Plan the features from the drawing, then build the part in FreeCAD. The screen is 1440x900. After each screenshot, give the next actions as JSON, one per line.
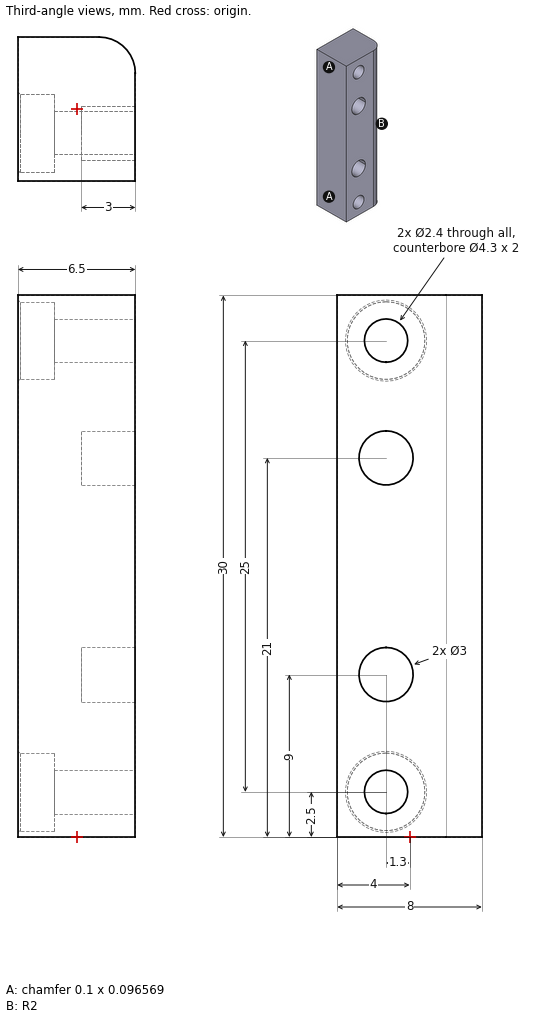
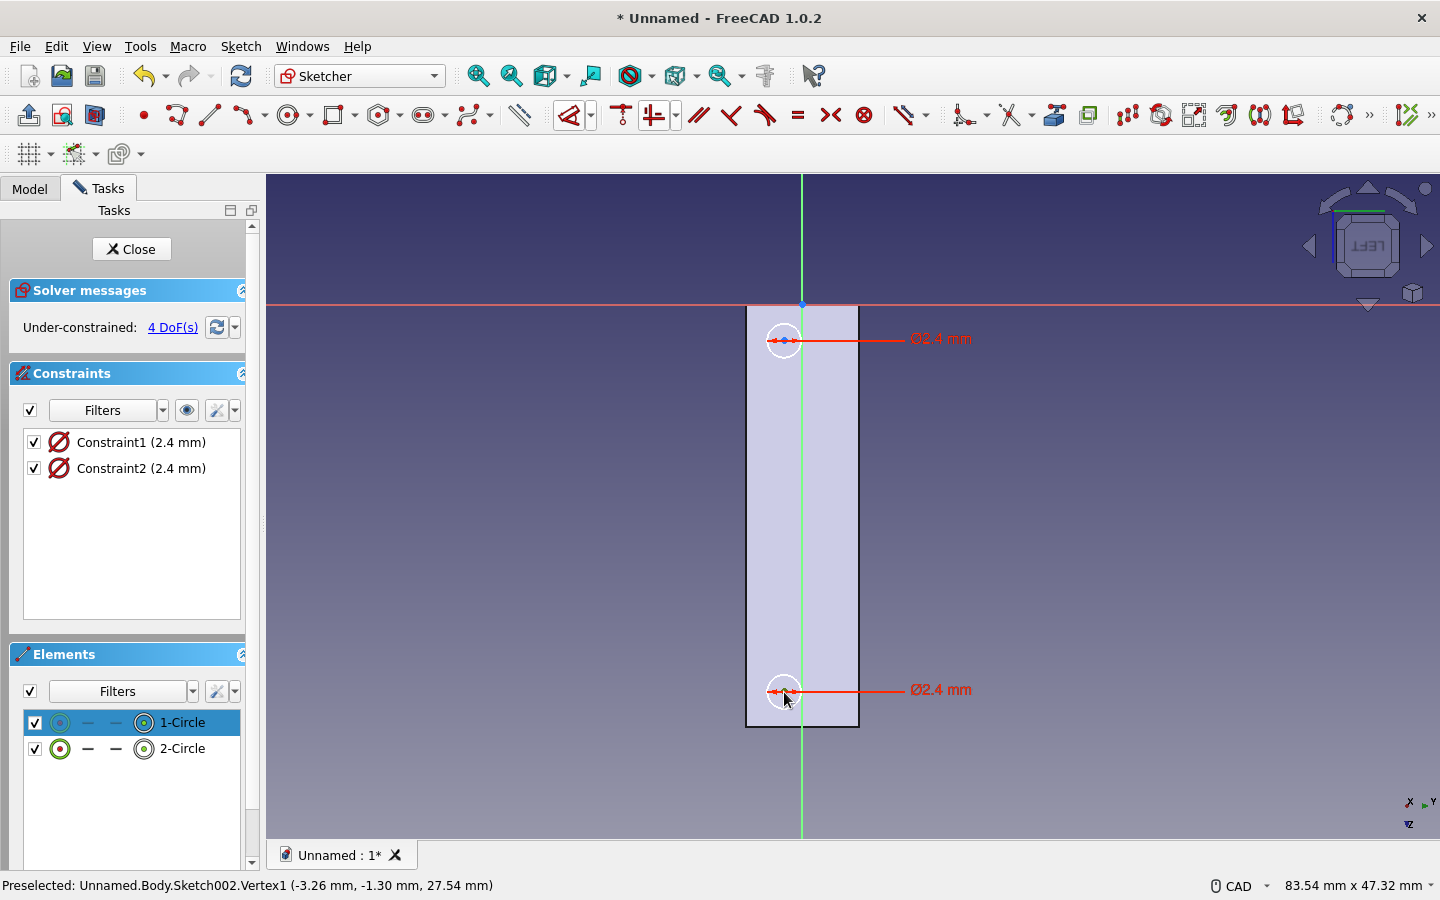
{"action": "left_click", "coordinate": [784, 341]}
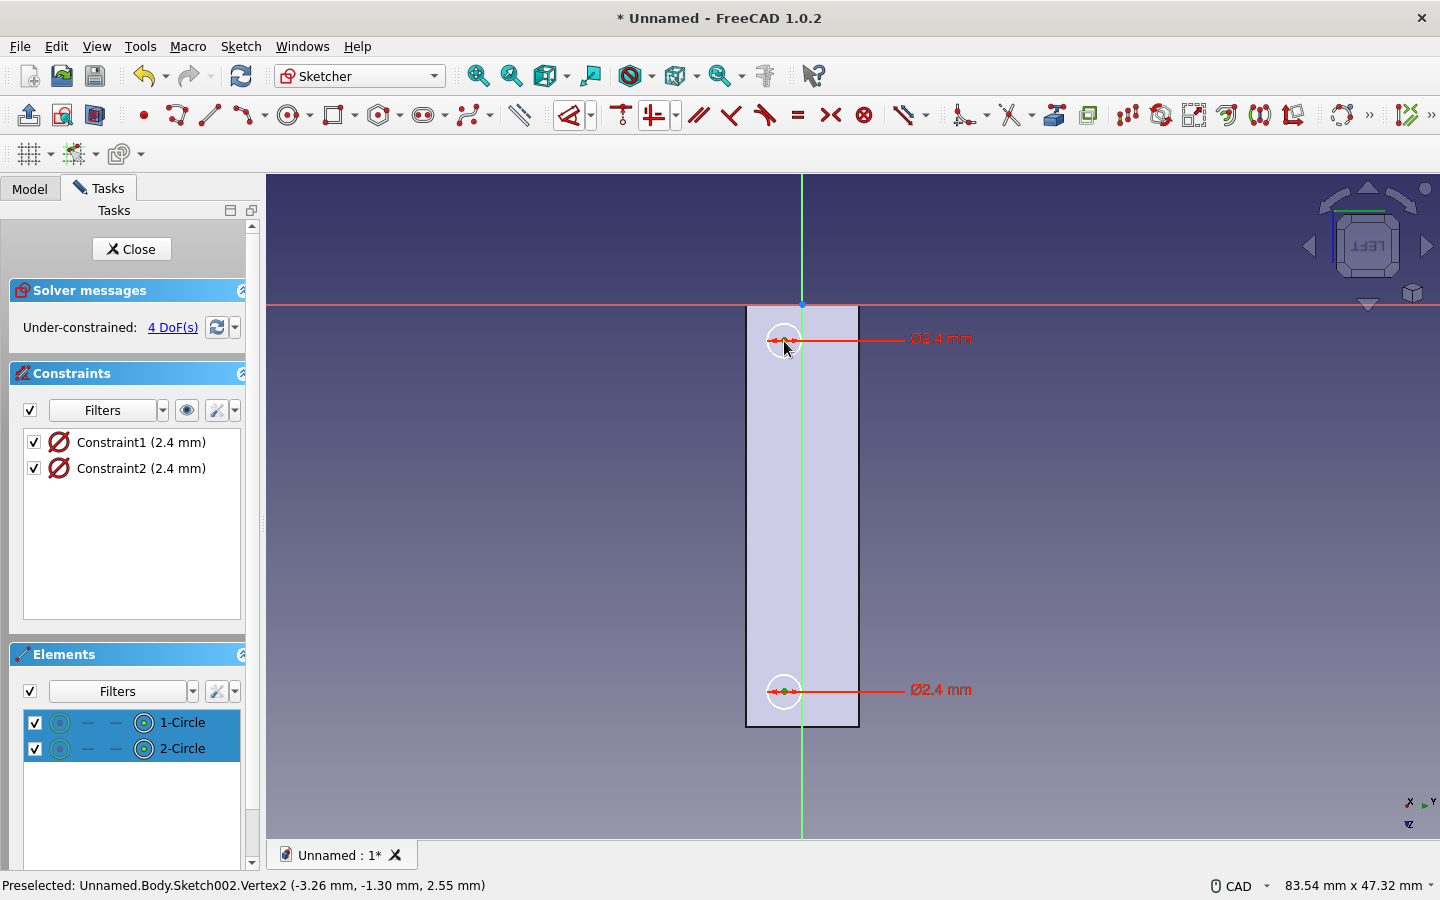
{"action": "key", "text": "v"}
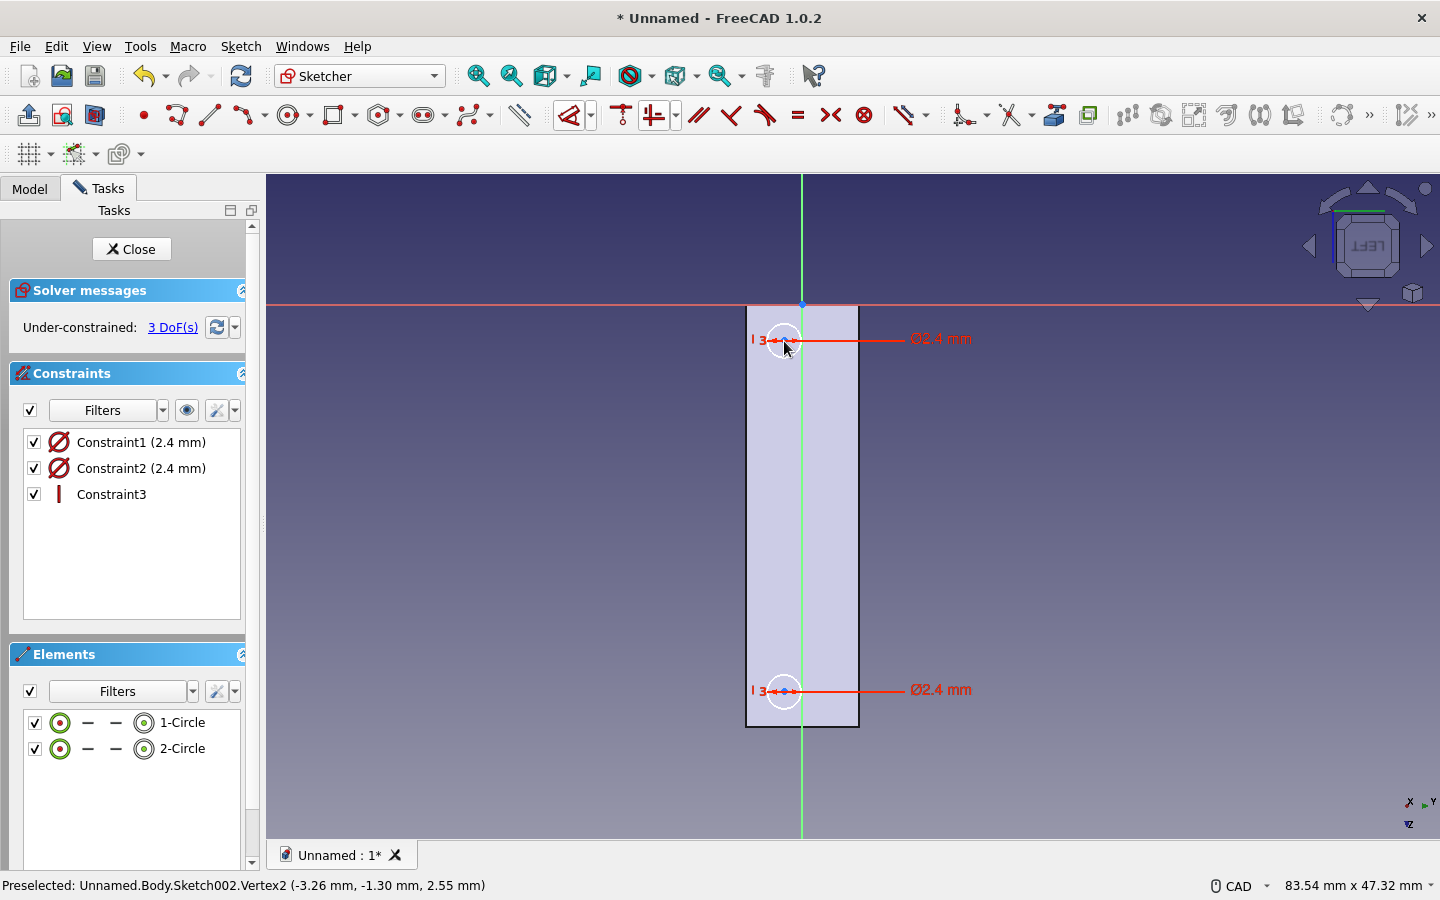
{"action": "scroll", "coordinate": [784, 692], "scroll_direction": "up", "scroll_amount": 4}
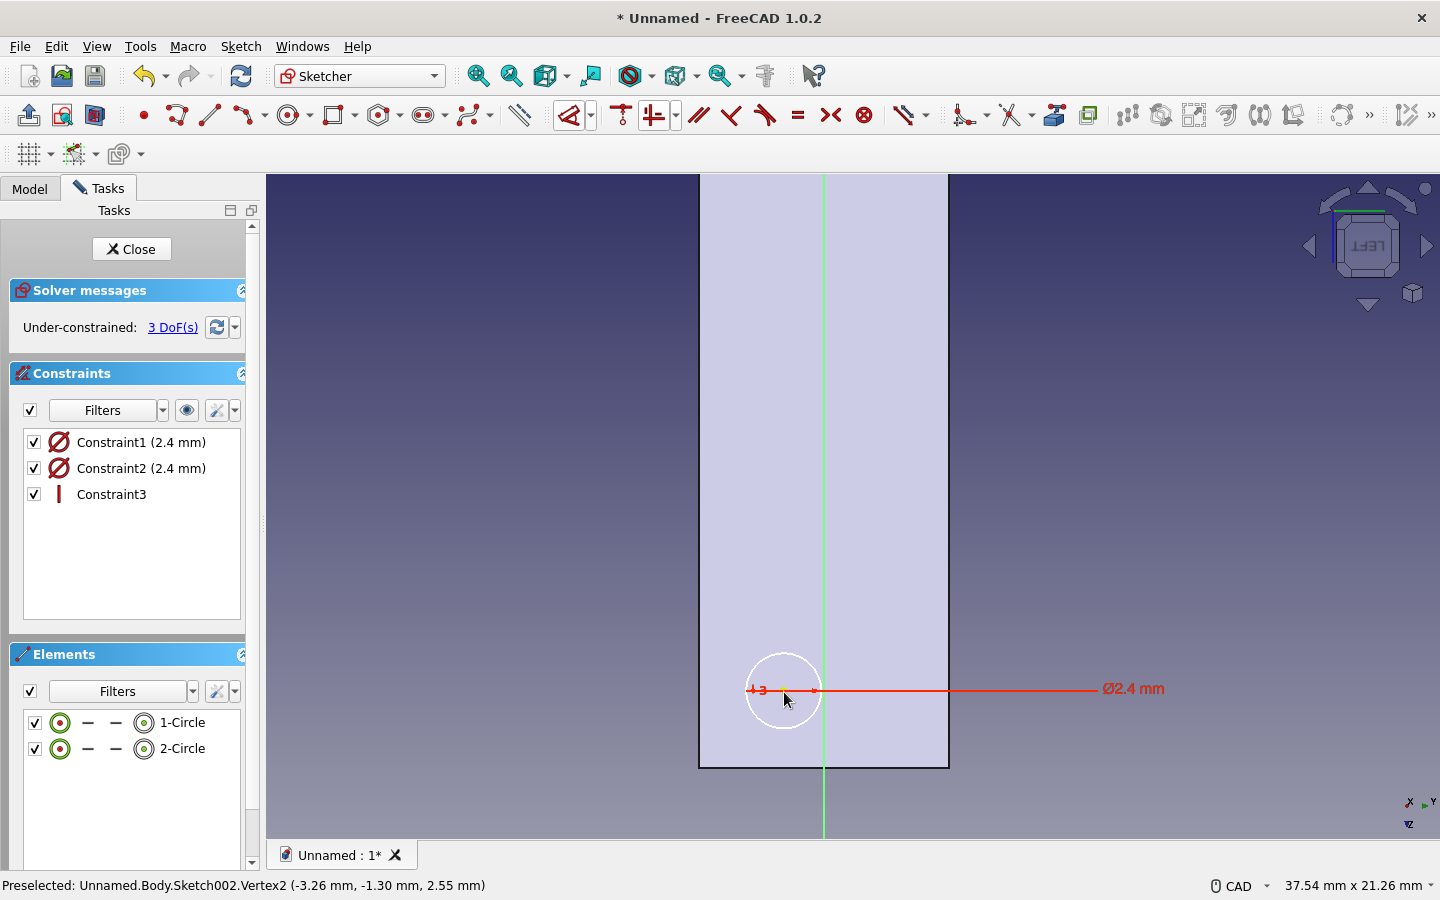
{"action": "left_click", "coordinate": [784, 691]}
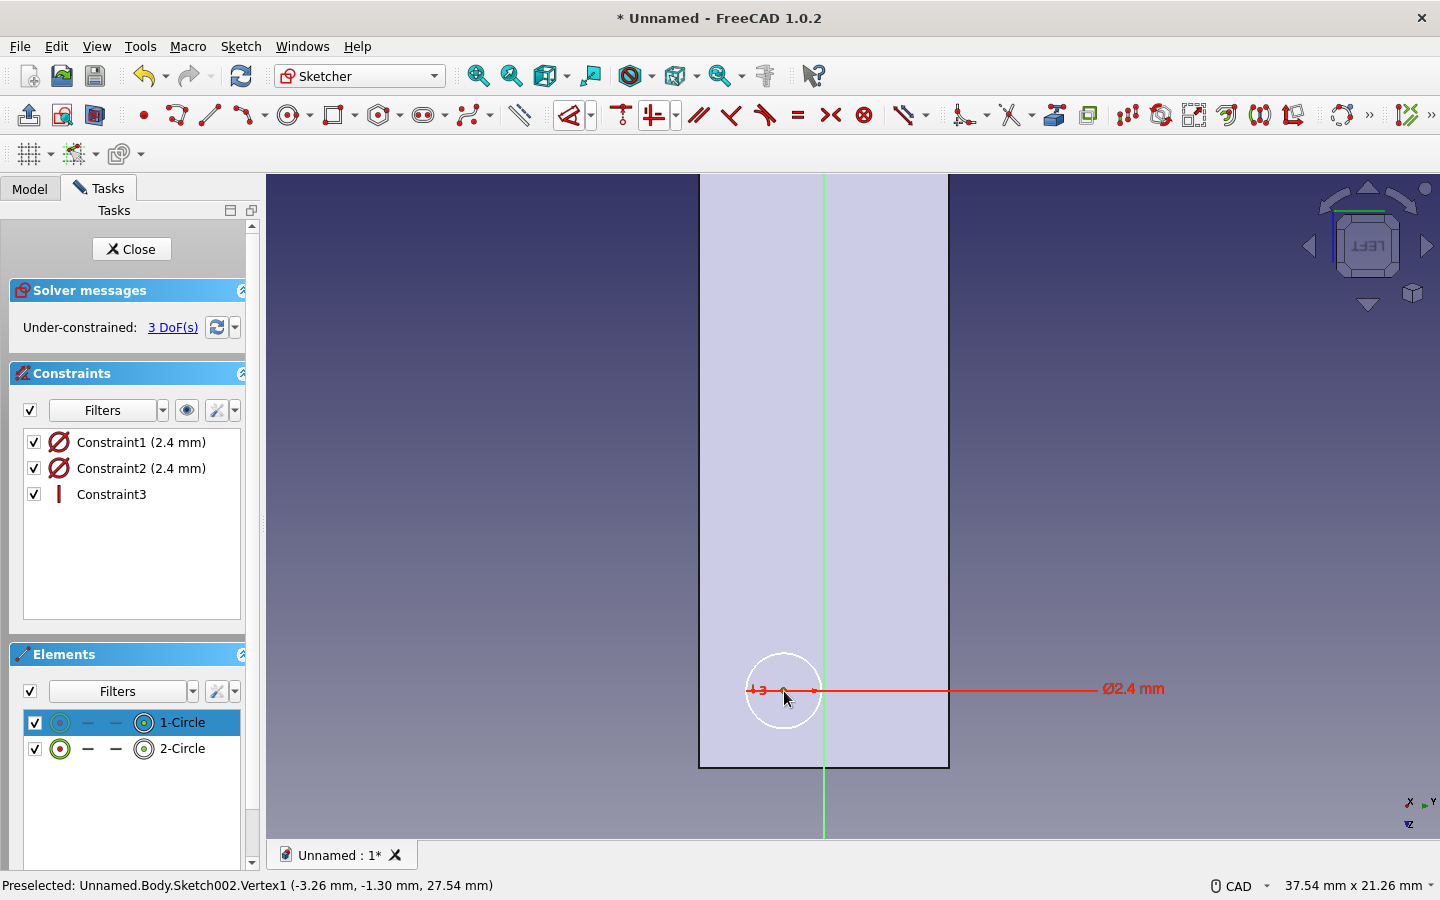
{"action": "left_click", "coordinate": [590, 116]}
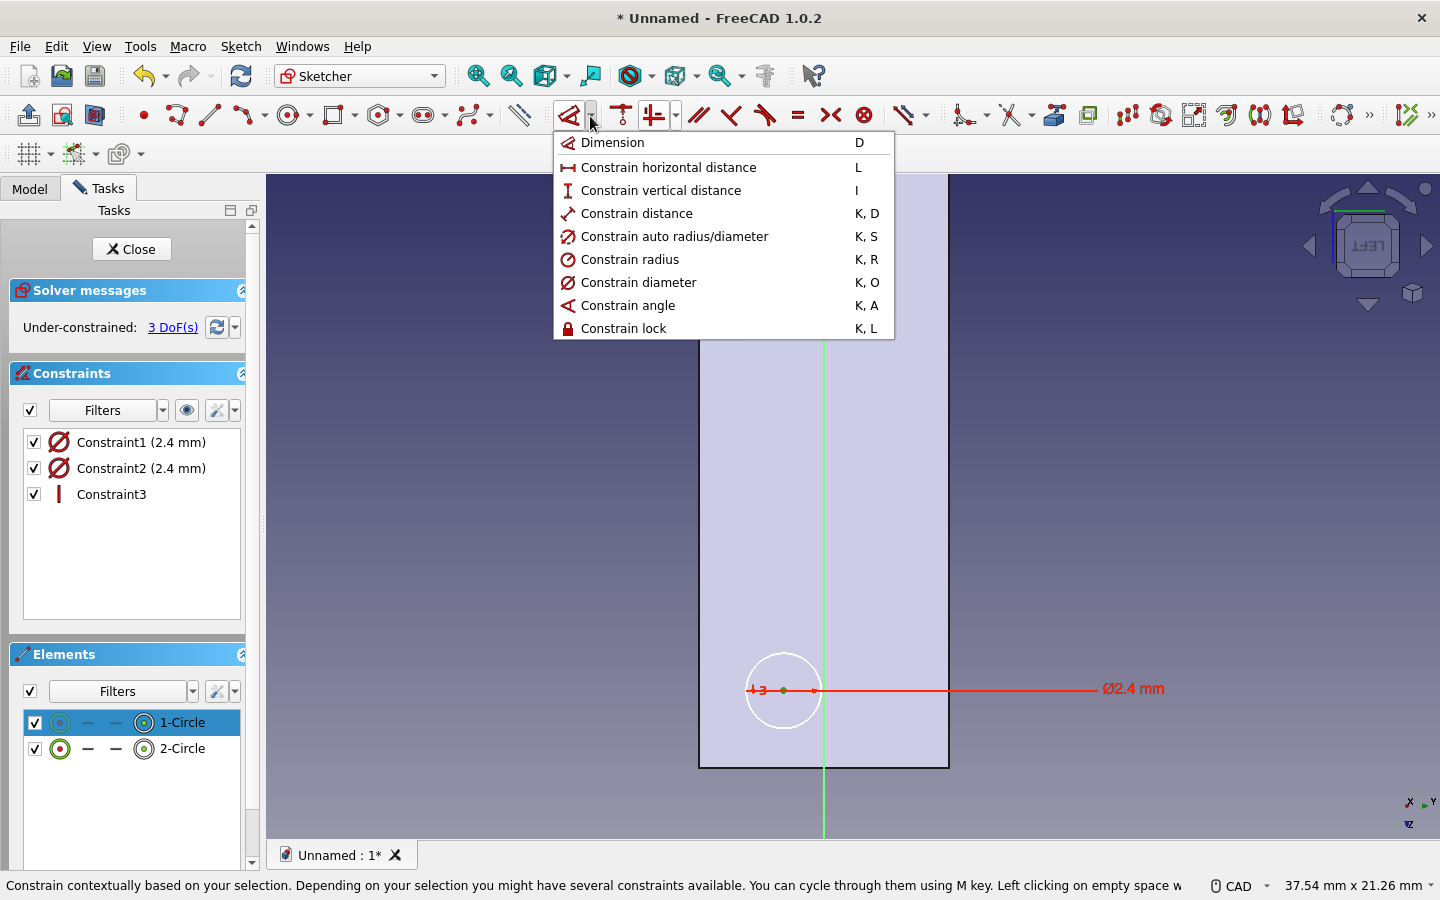
{"action": "left_click", "coordinate": [724, 168]}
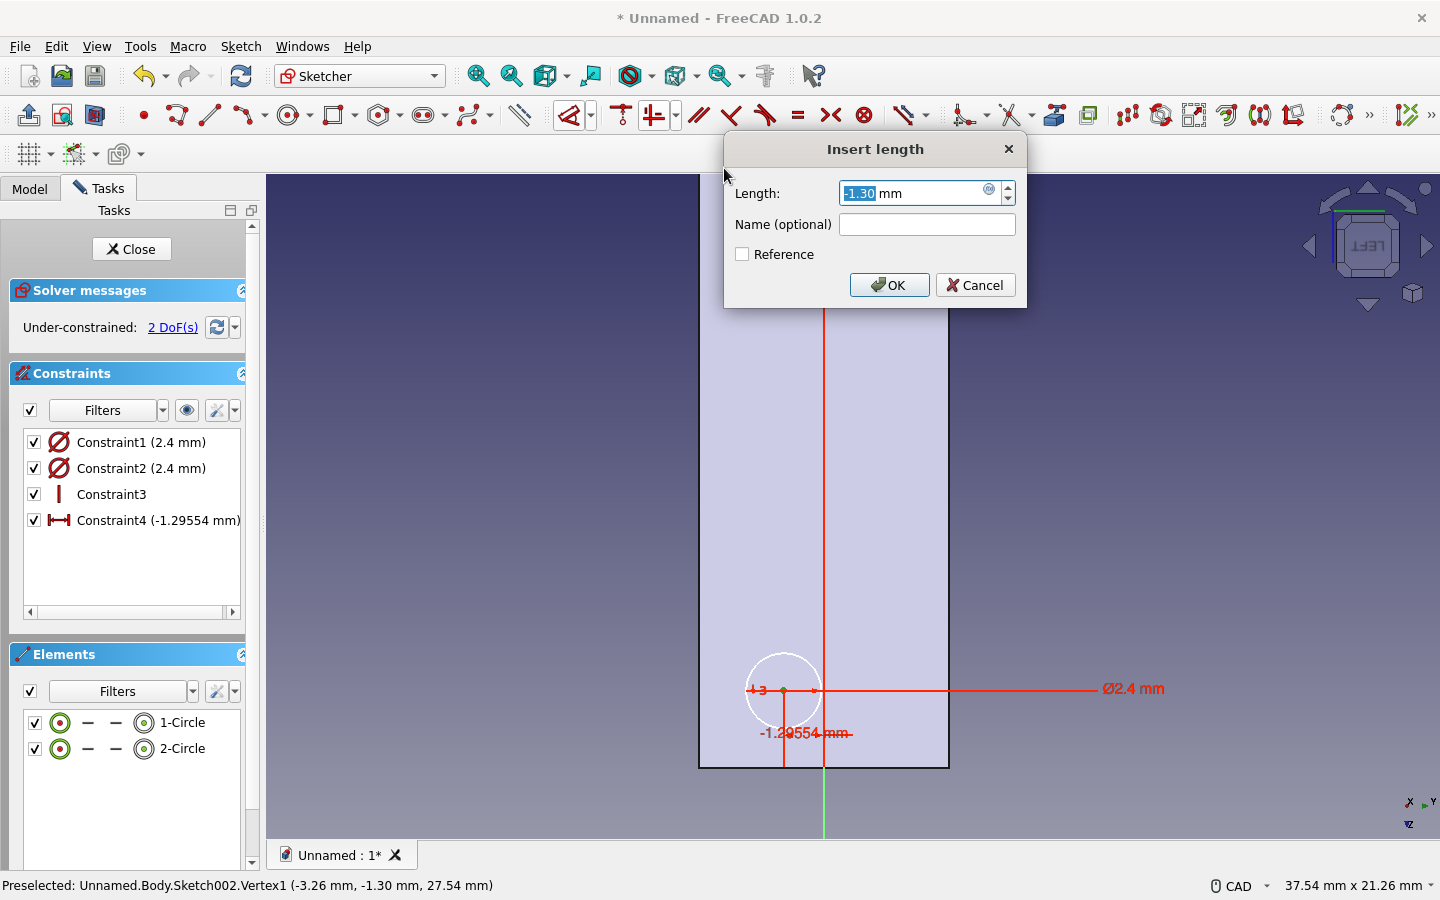
{"action": "type", "text": "-1.3"}
{"action": "key", "text": "Return"}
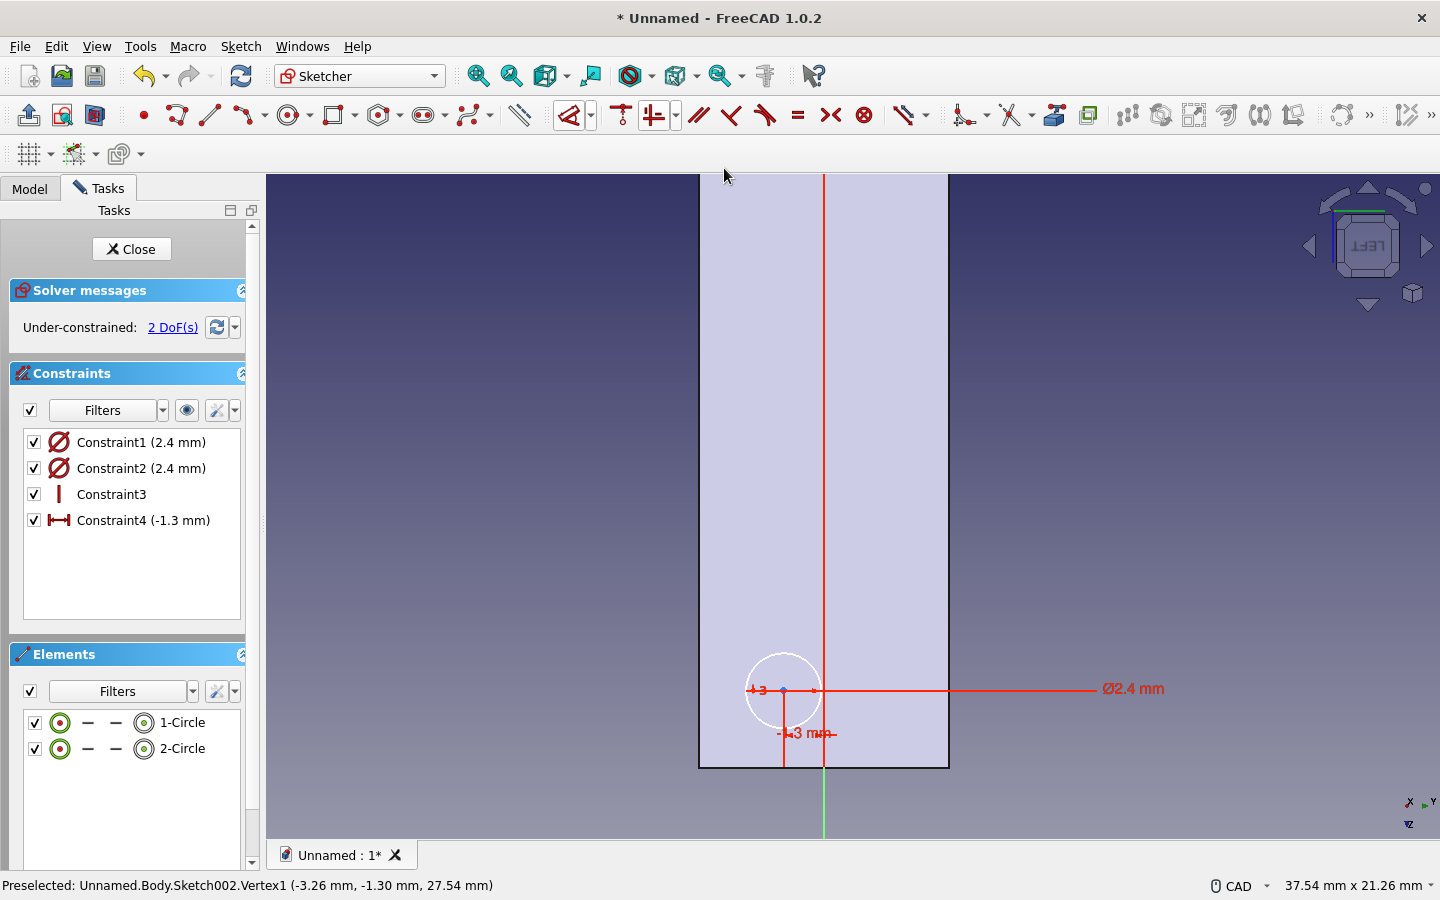
{"action": "scroll", "coordinate": [784, 693], "scroll_direction": "down", "scroll_amount": 4}